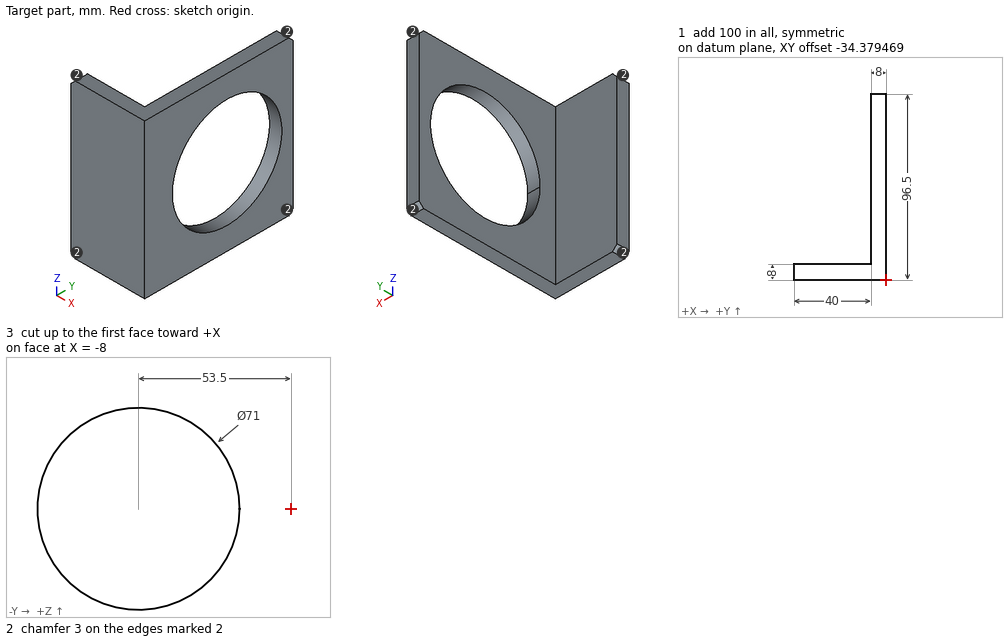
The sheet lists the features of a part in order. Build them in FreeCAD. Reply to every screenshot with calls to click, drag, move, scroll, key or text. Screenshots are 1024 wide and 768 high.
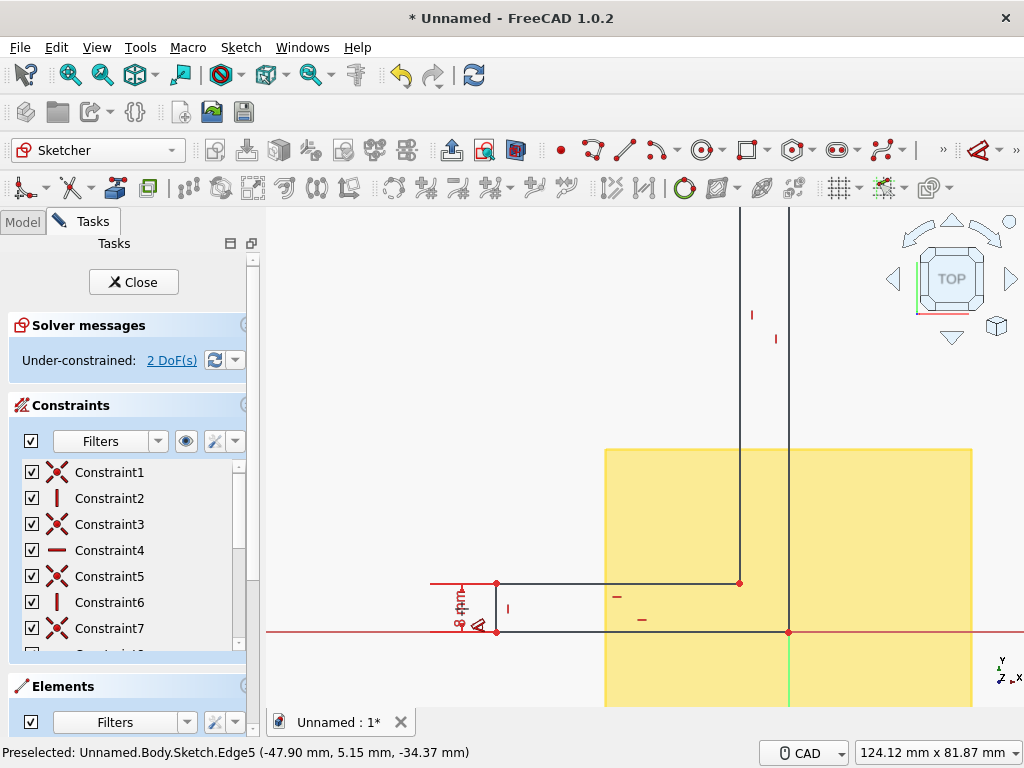
click(667, 584)
click(618, 618)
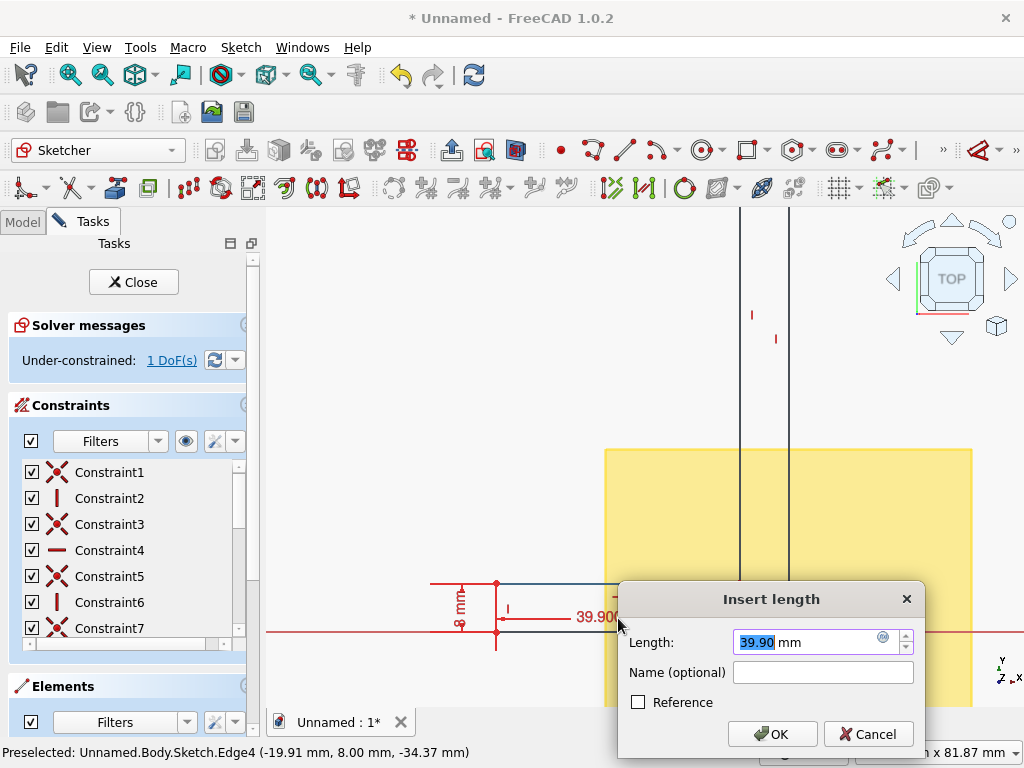
text(40)
key(Return)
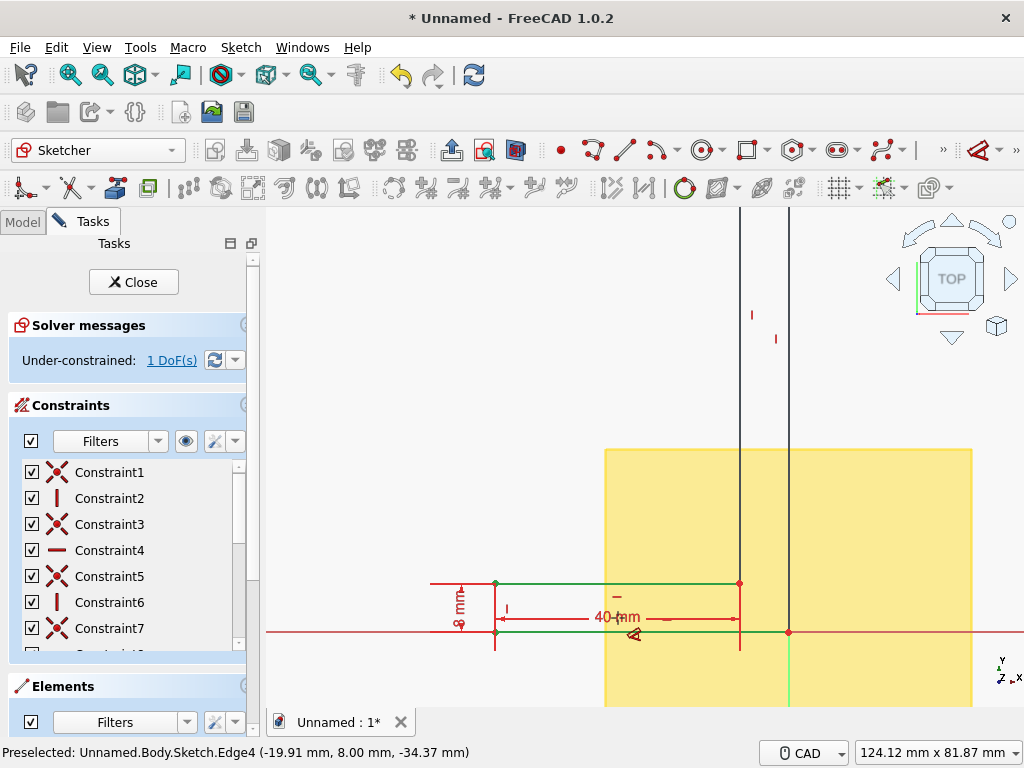
click(789, 456)
click(823, 434)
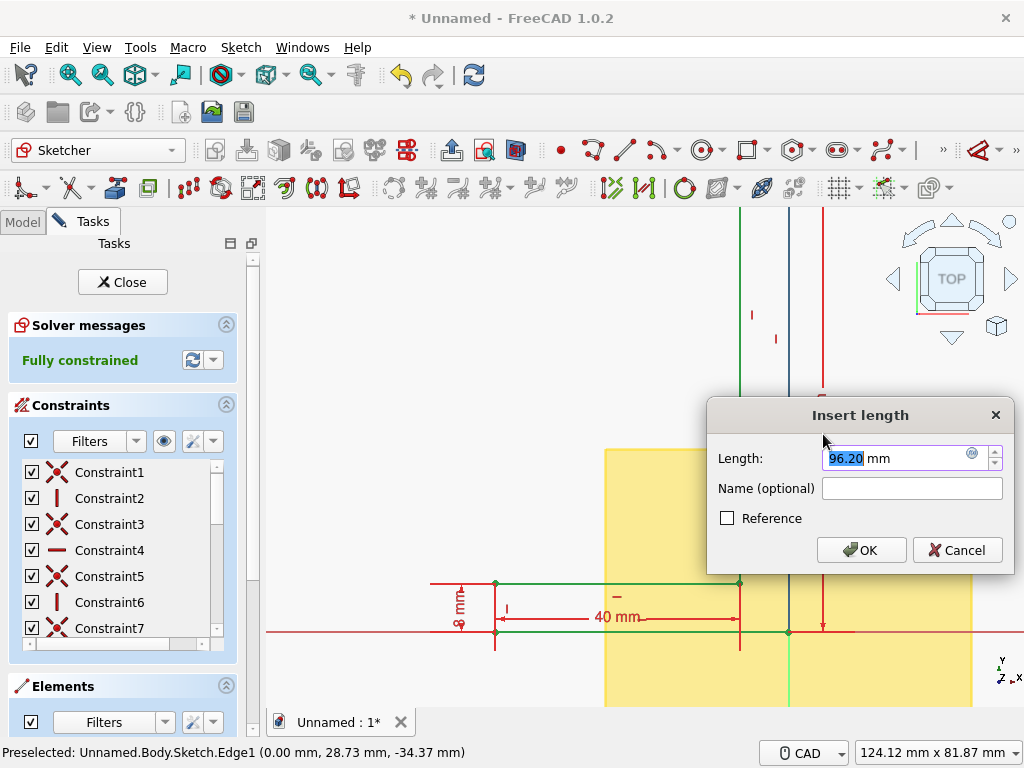
text(96.5)
key(Return)
key(Escape)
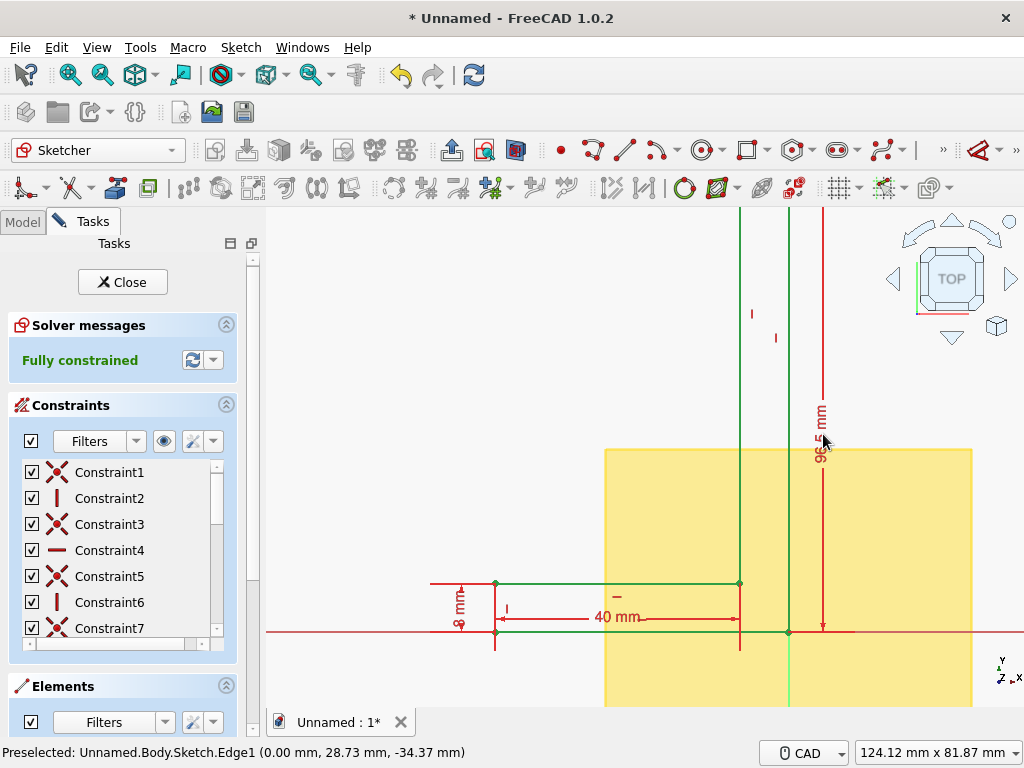
click(123, 282)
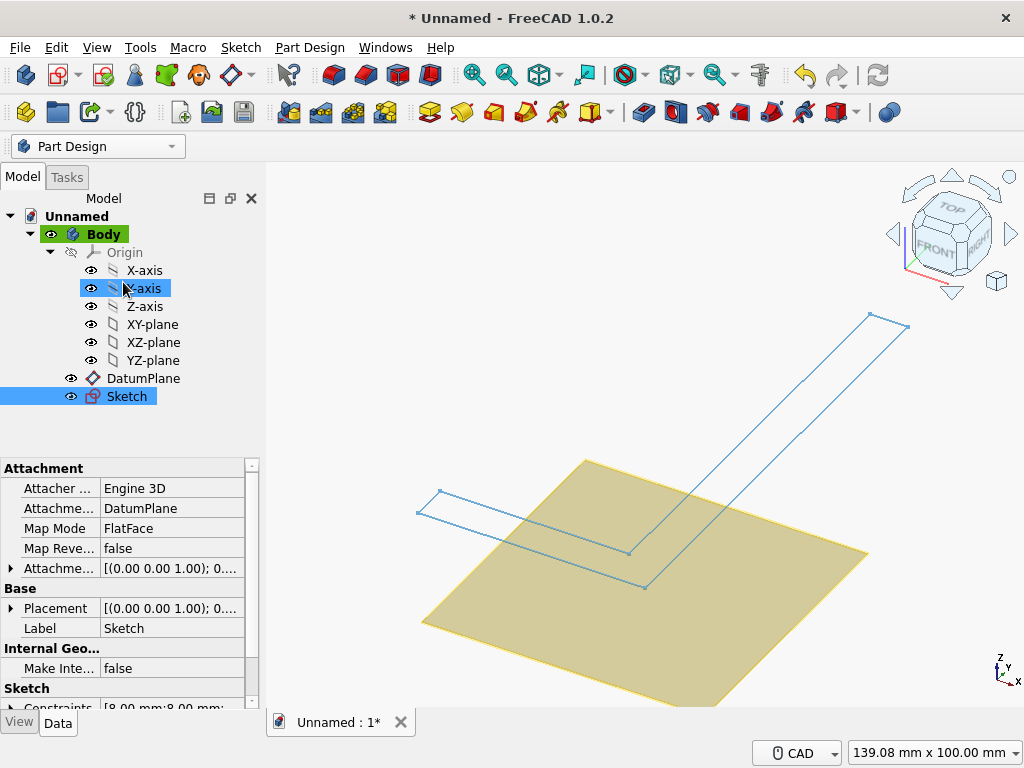
click(430, 112)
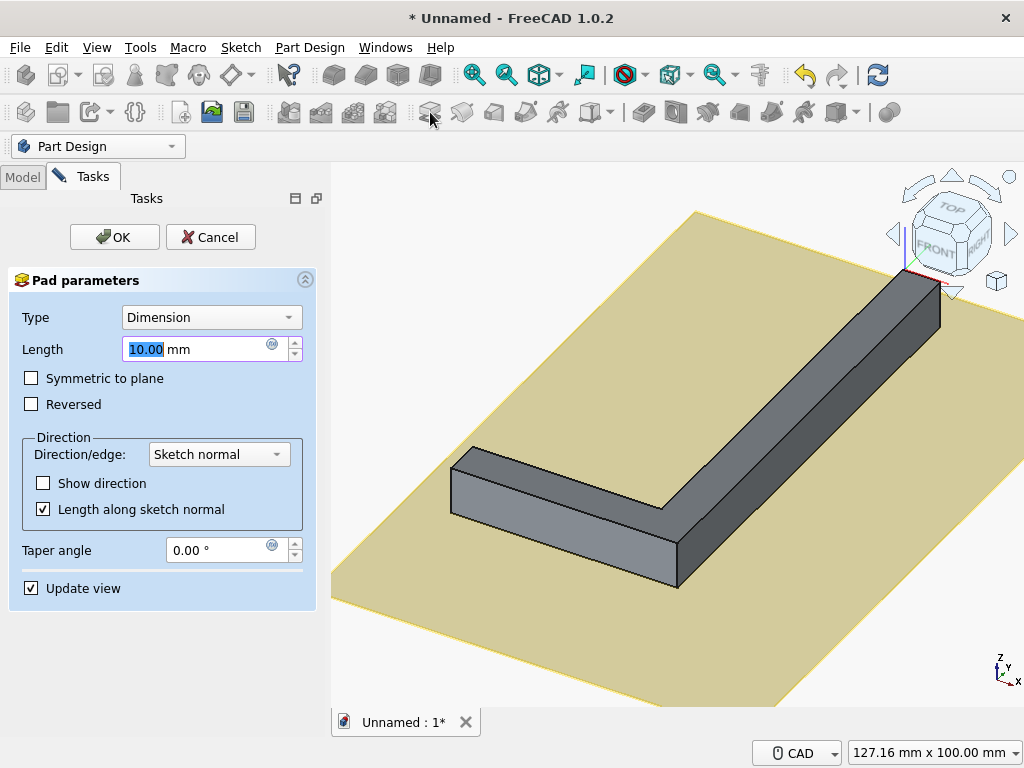
text(100)
key(Tab)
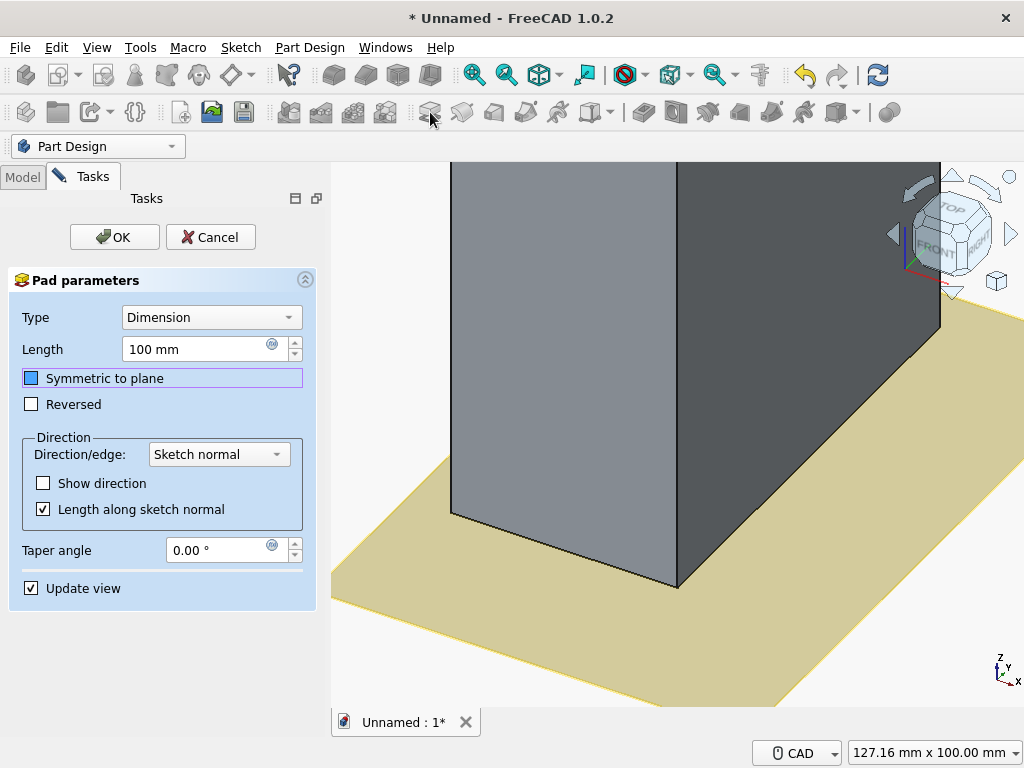
click(30, 378)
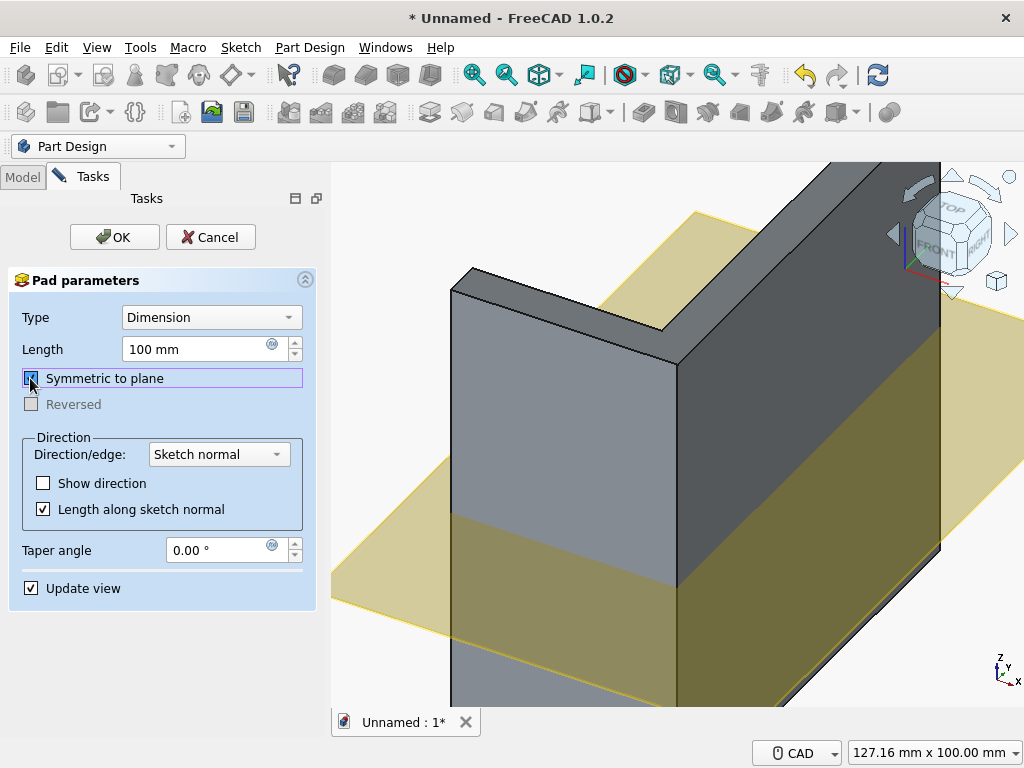
click(115, 237)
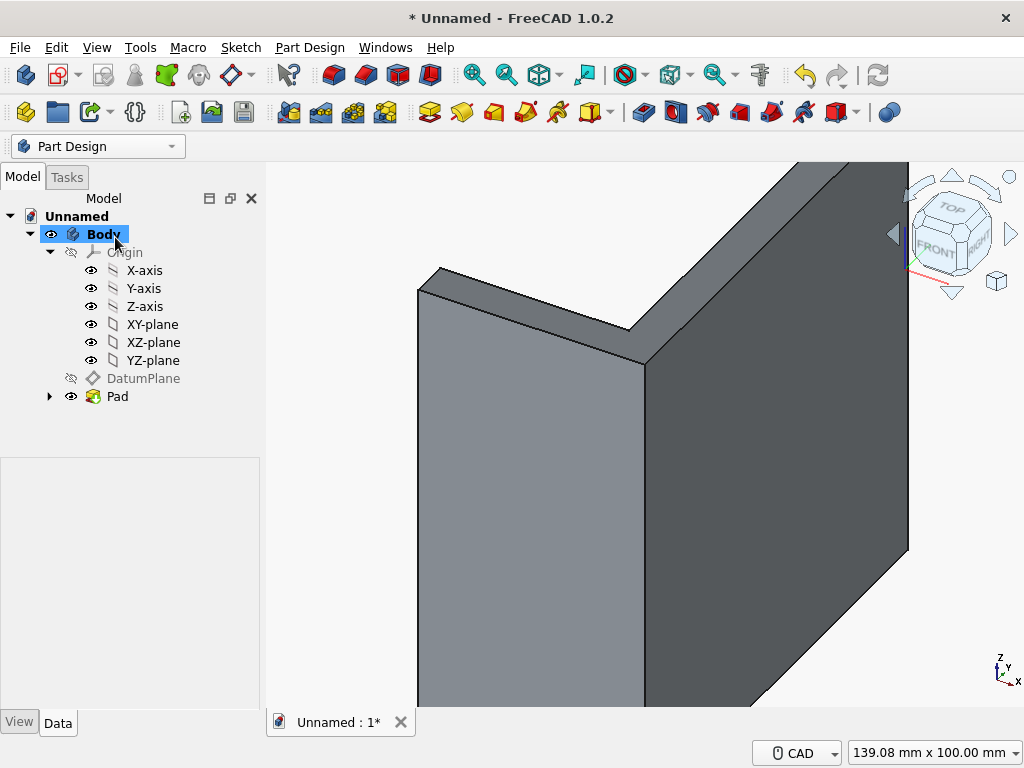
key(v)
key(f)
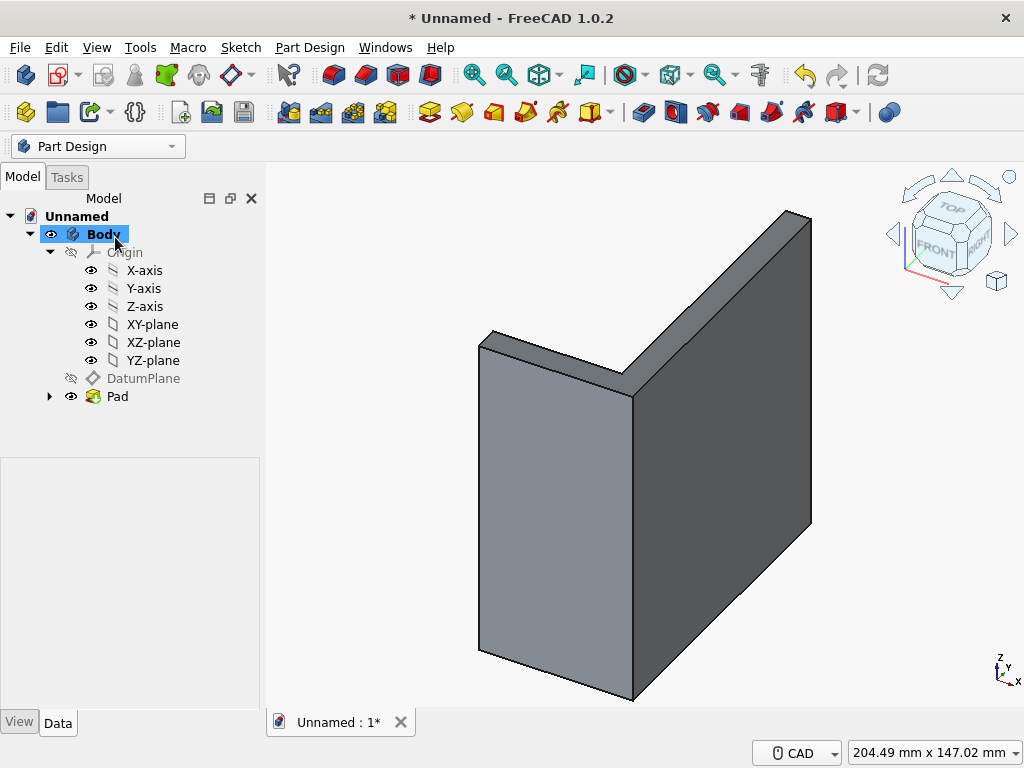
key(0)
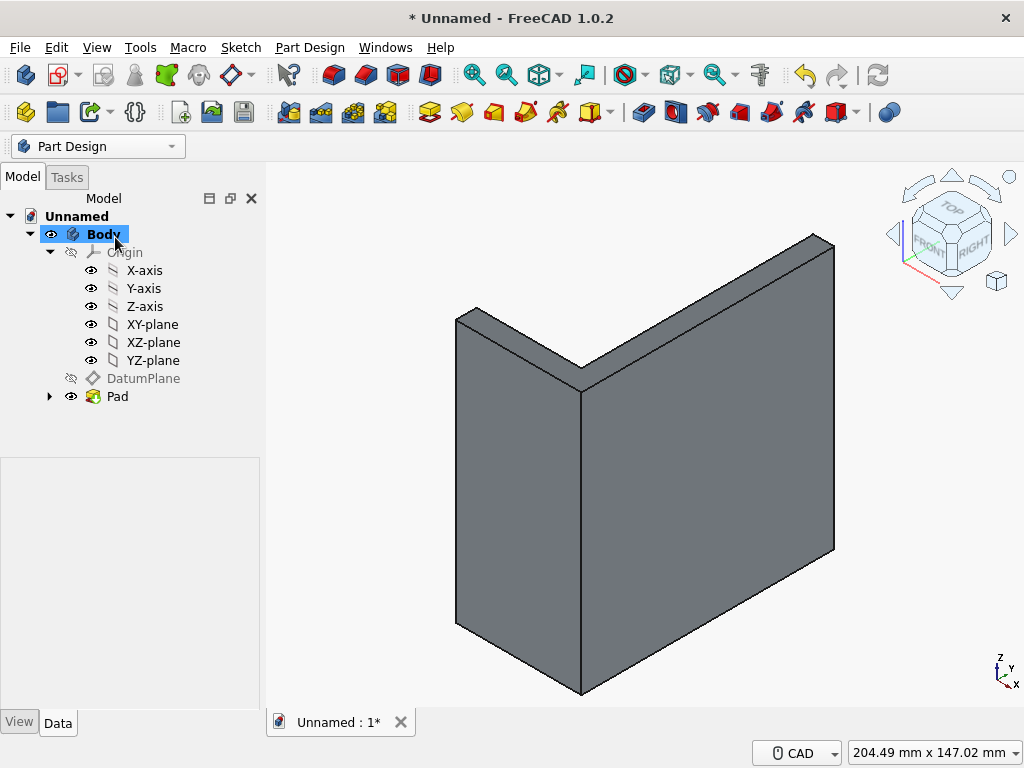
key(2)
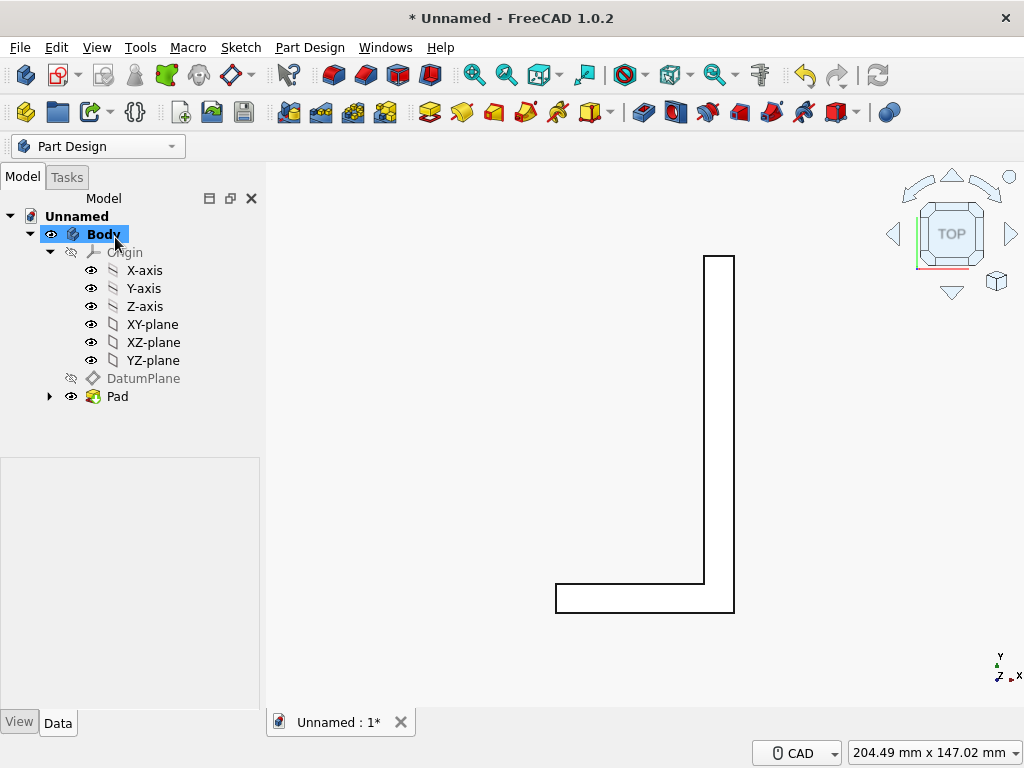
click(556, 598)